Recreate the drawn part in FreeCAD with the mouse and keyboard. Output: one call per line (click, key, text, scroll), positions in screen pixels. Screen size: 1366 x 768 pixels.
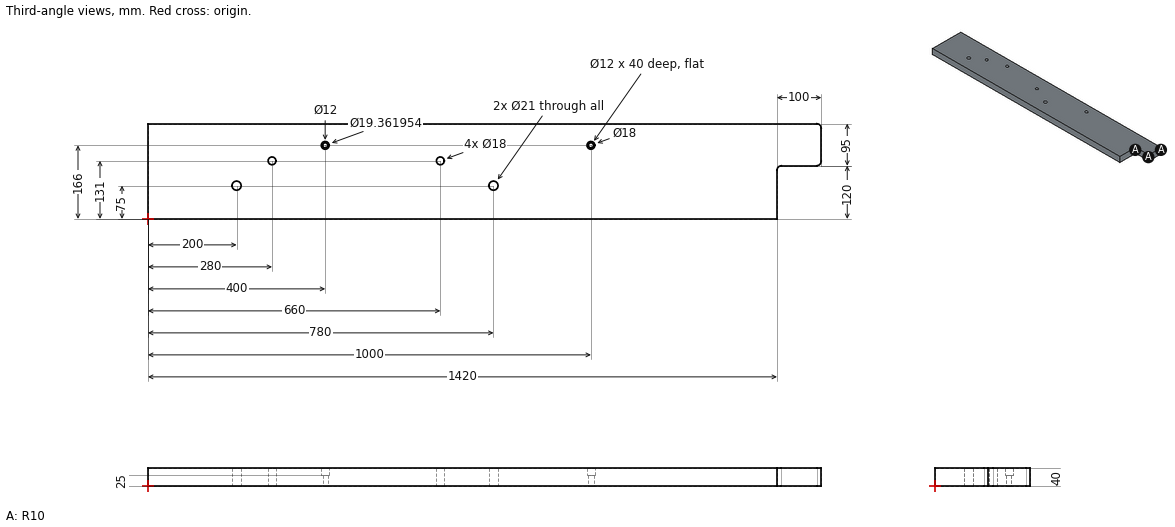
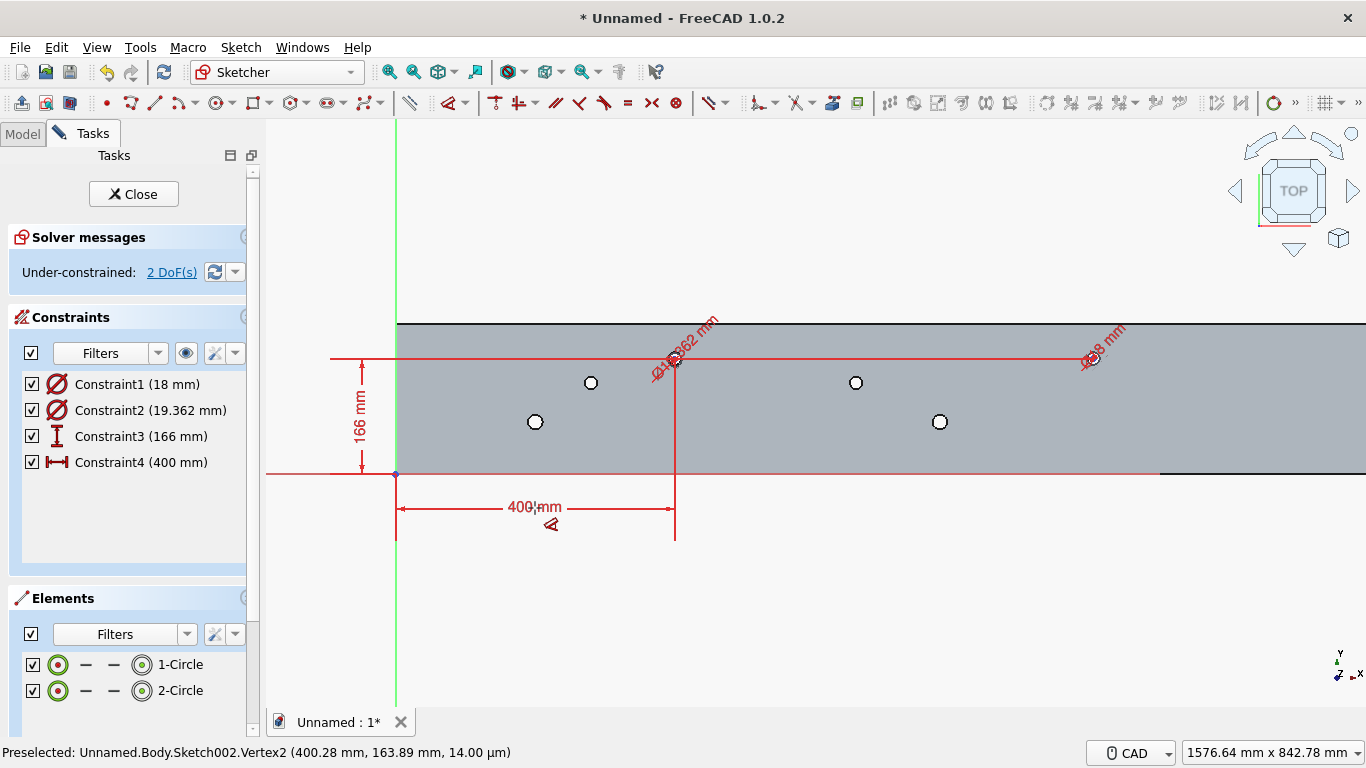
click(675, 360)
click(362, 391)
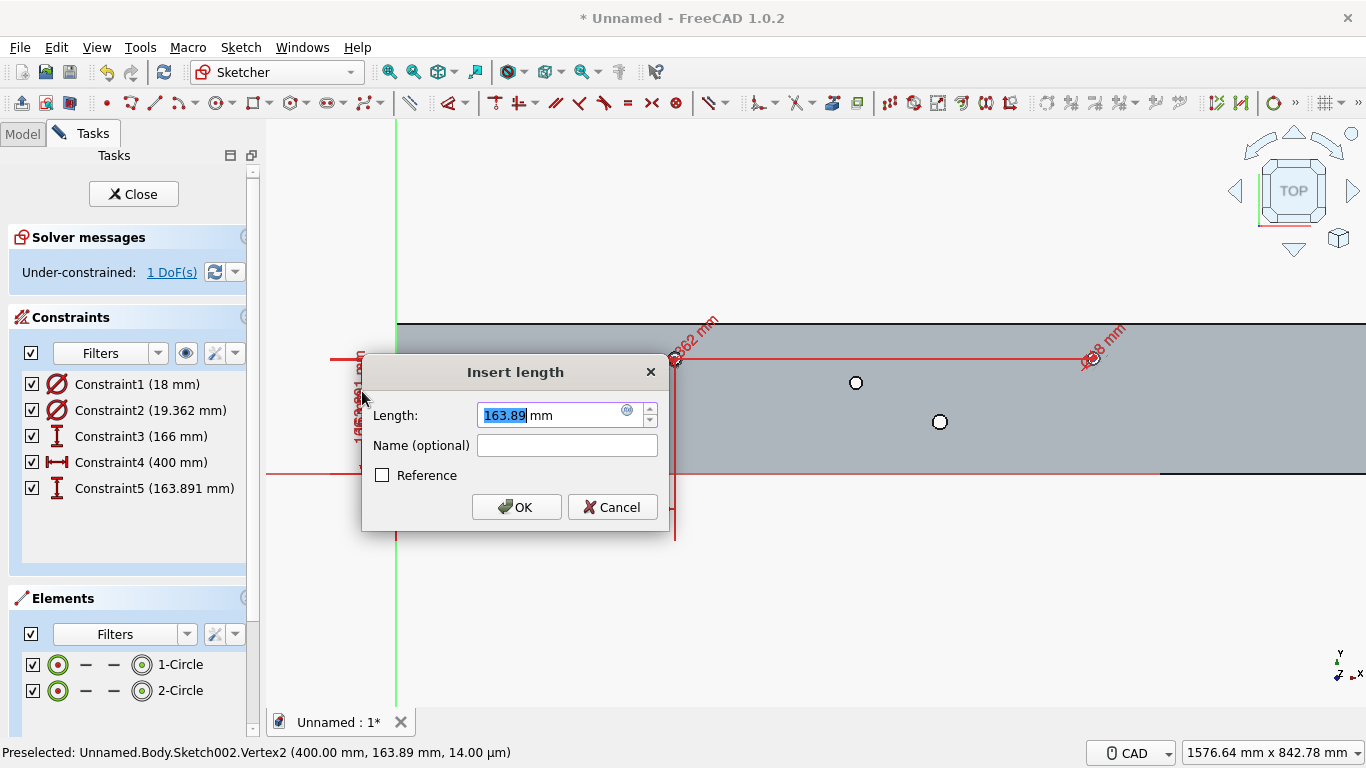
text(166)
key(Return)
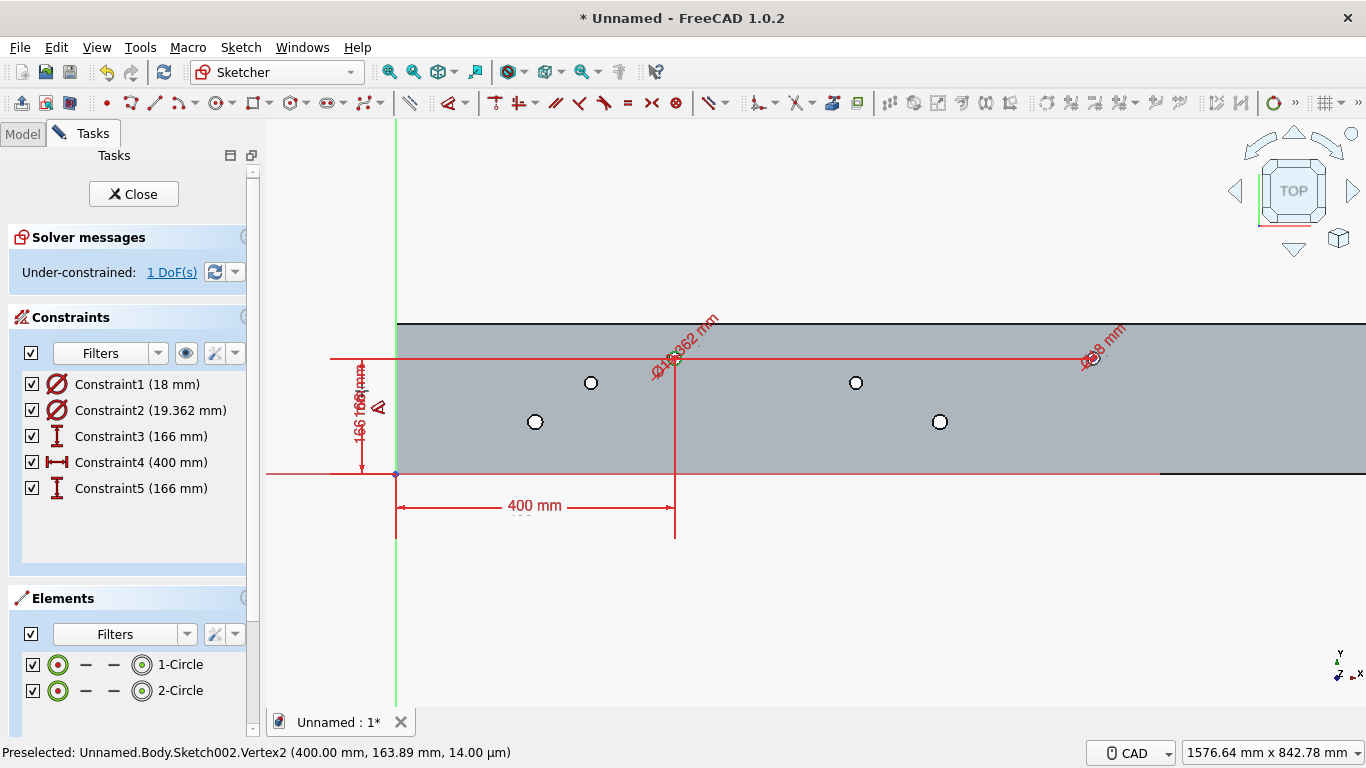
click(1093, 359)
click(745, 508)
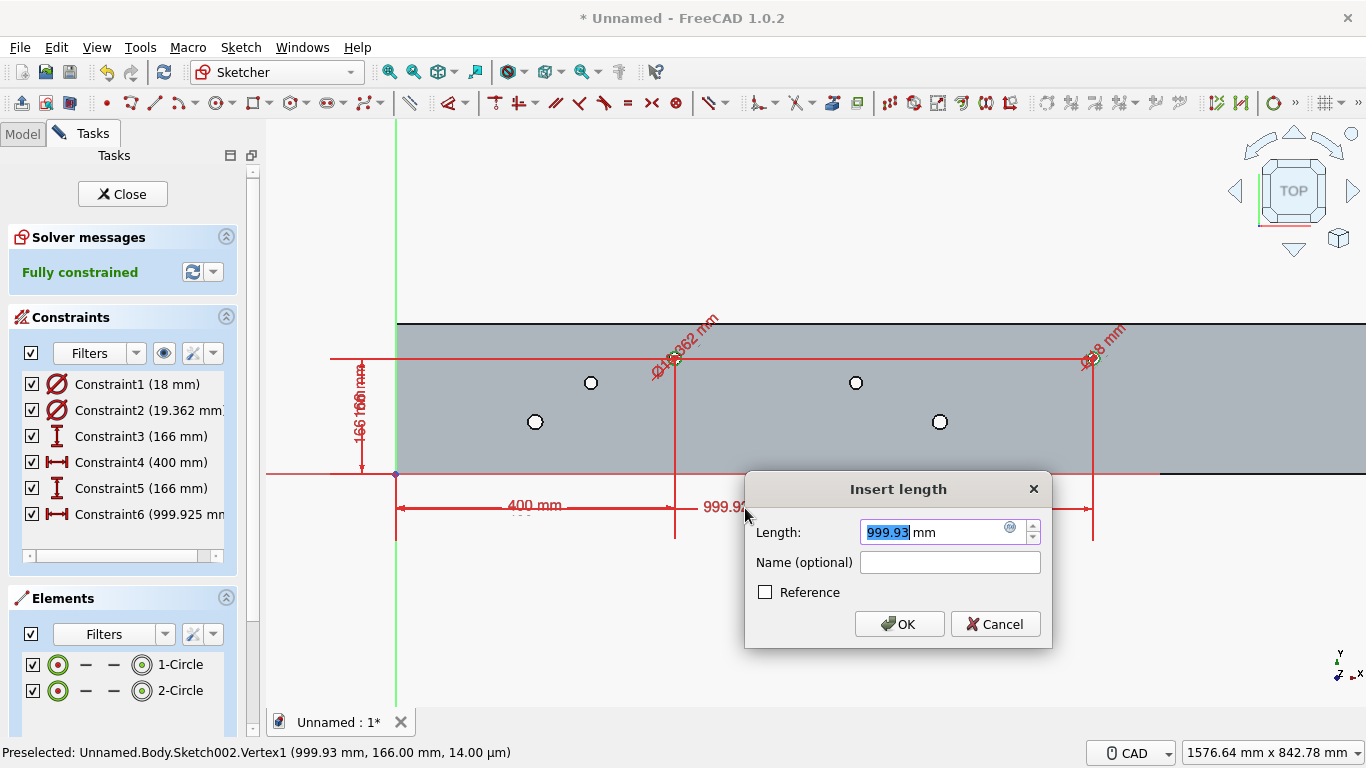
text(1000)
key(Return)
key(Escape)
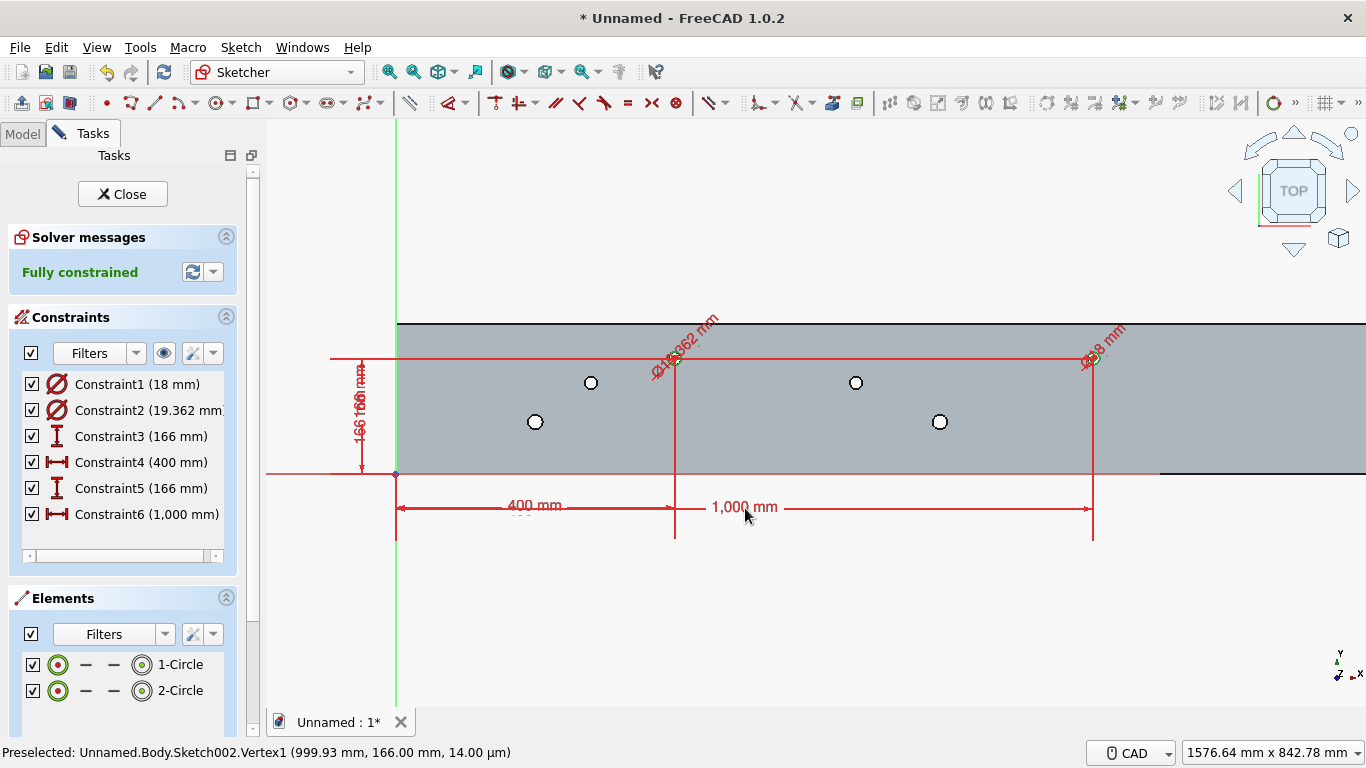
click(123, 194)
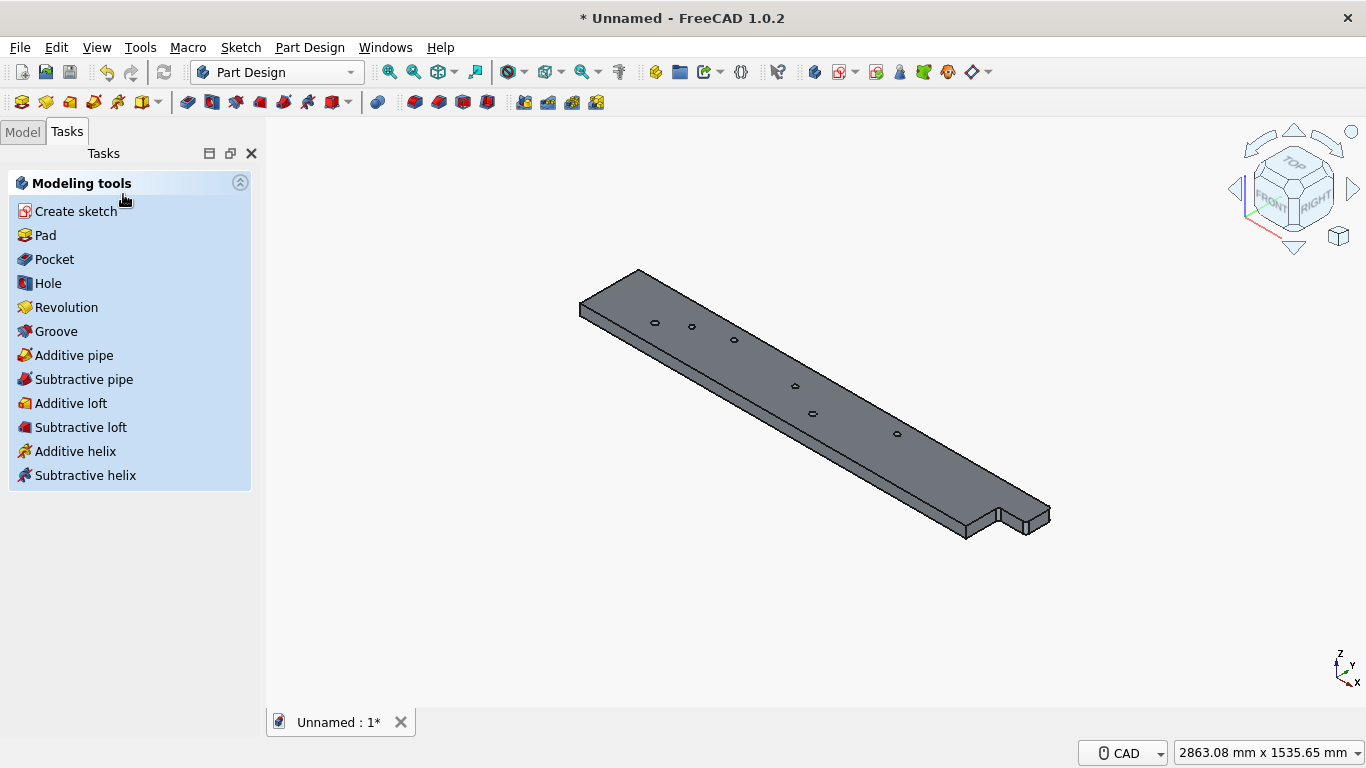
click(22, 102)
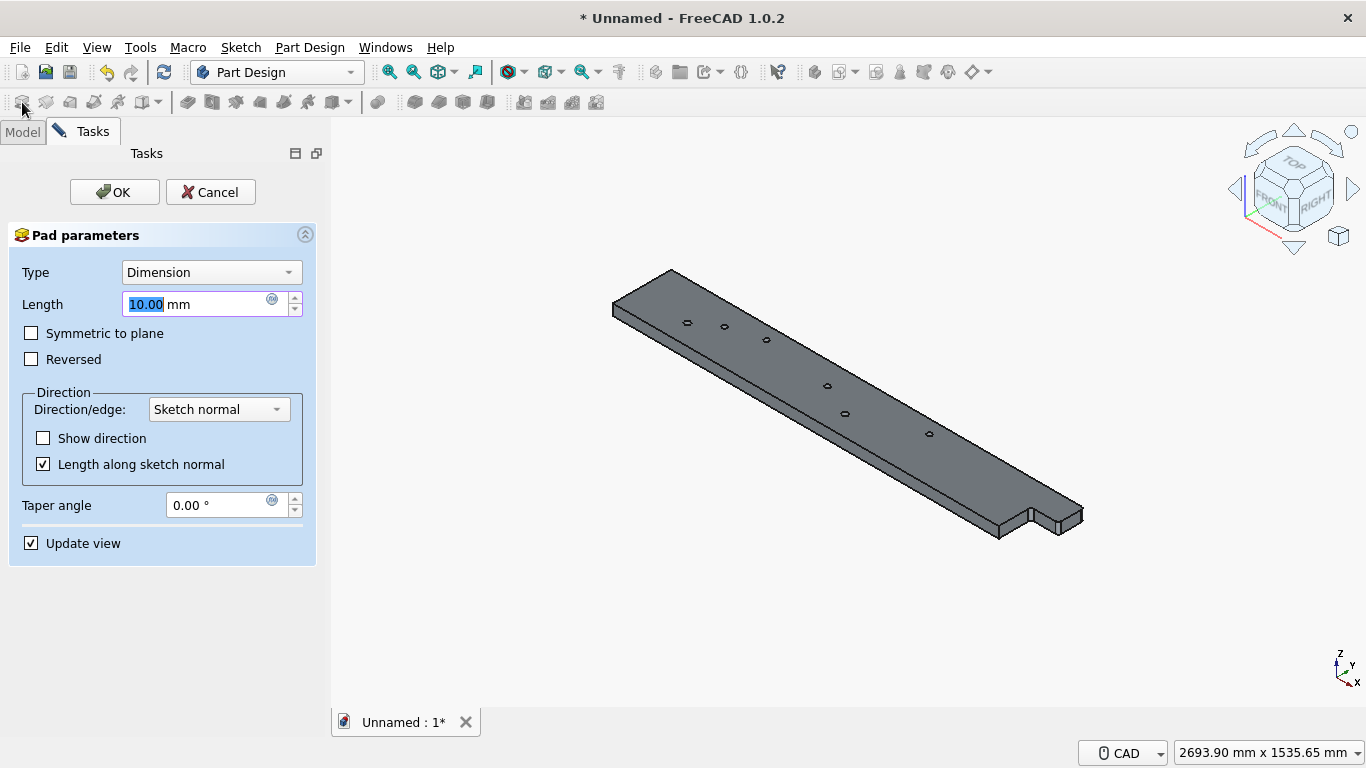
text(25)
key(Tab)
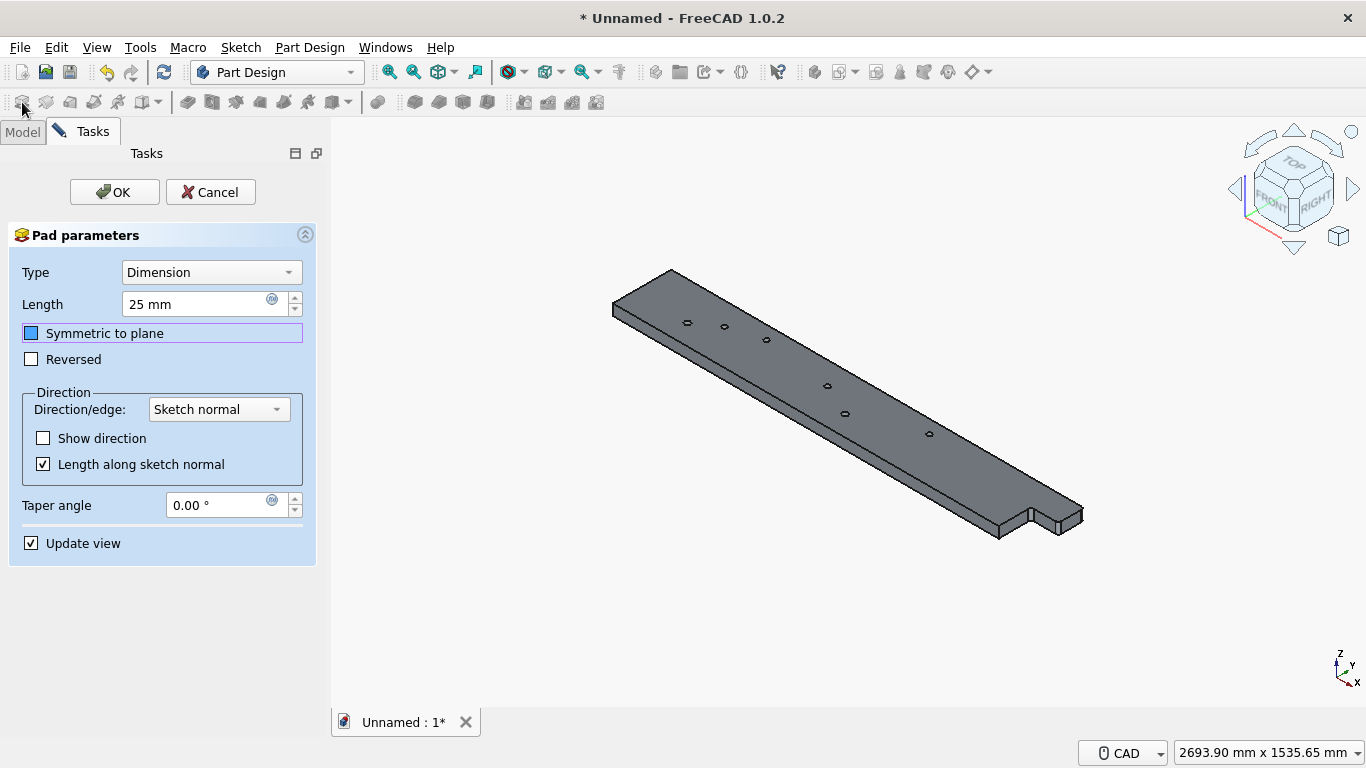
click(115, 192)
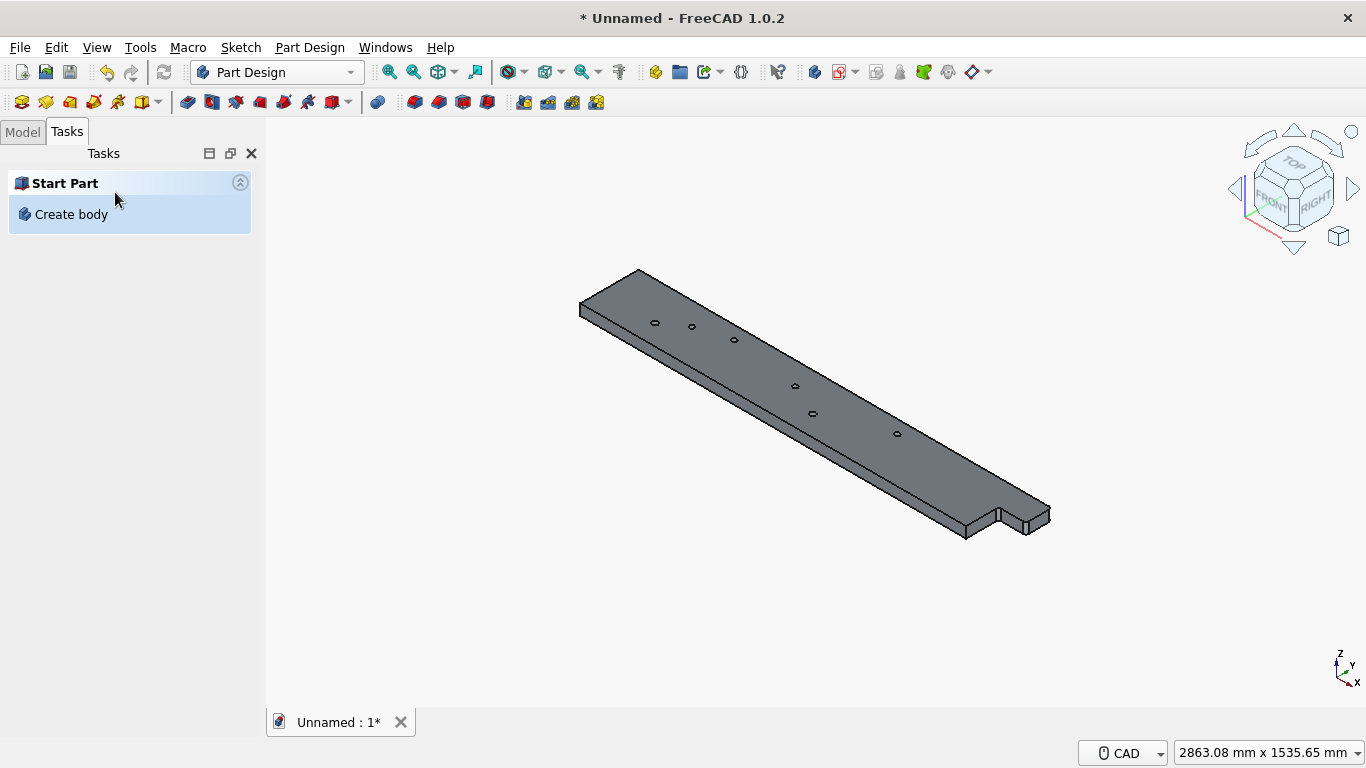
click(934, 473)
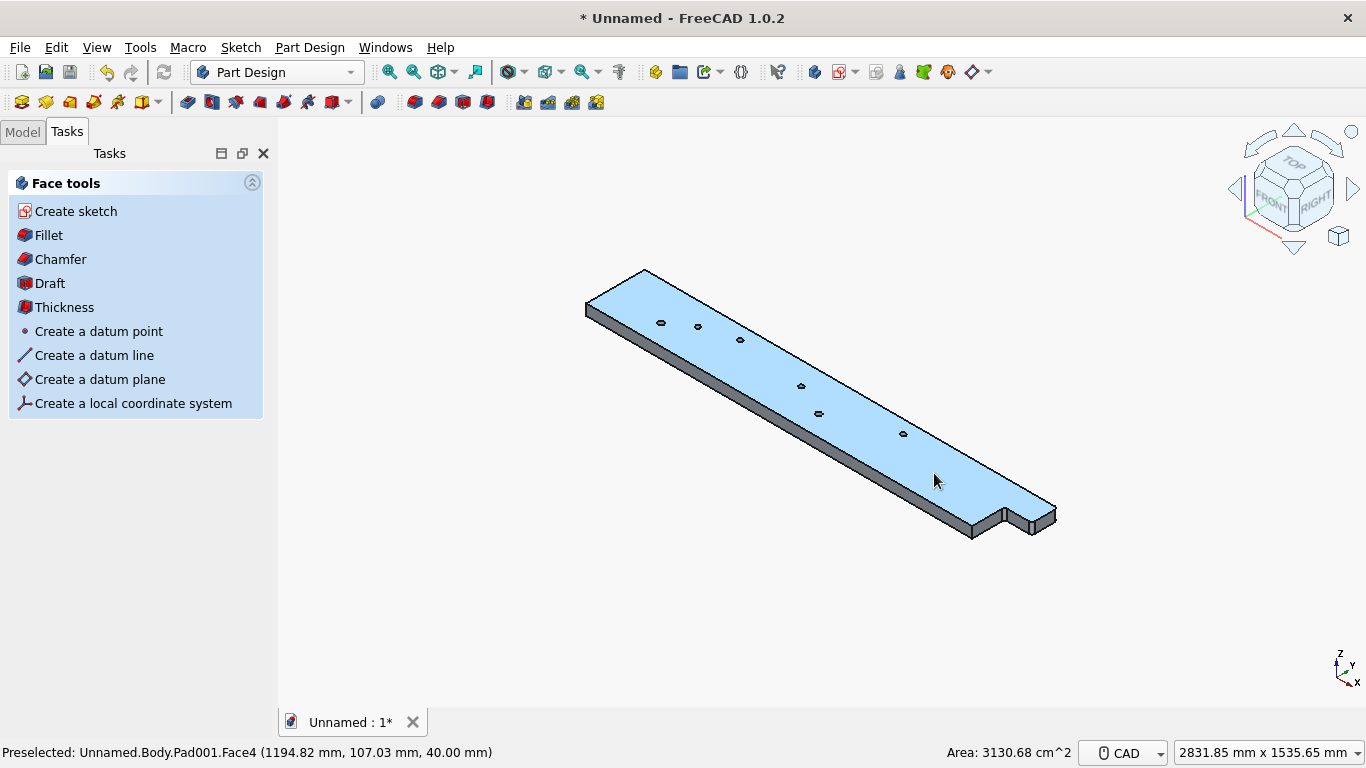
click(840, 72)